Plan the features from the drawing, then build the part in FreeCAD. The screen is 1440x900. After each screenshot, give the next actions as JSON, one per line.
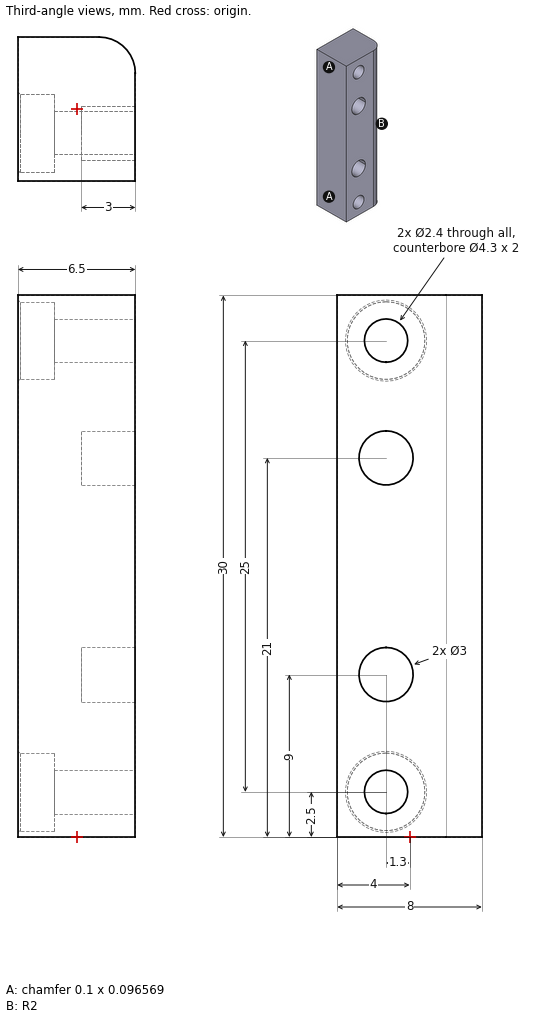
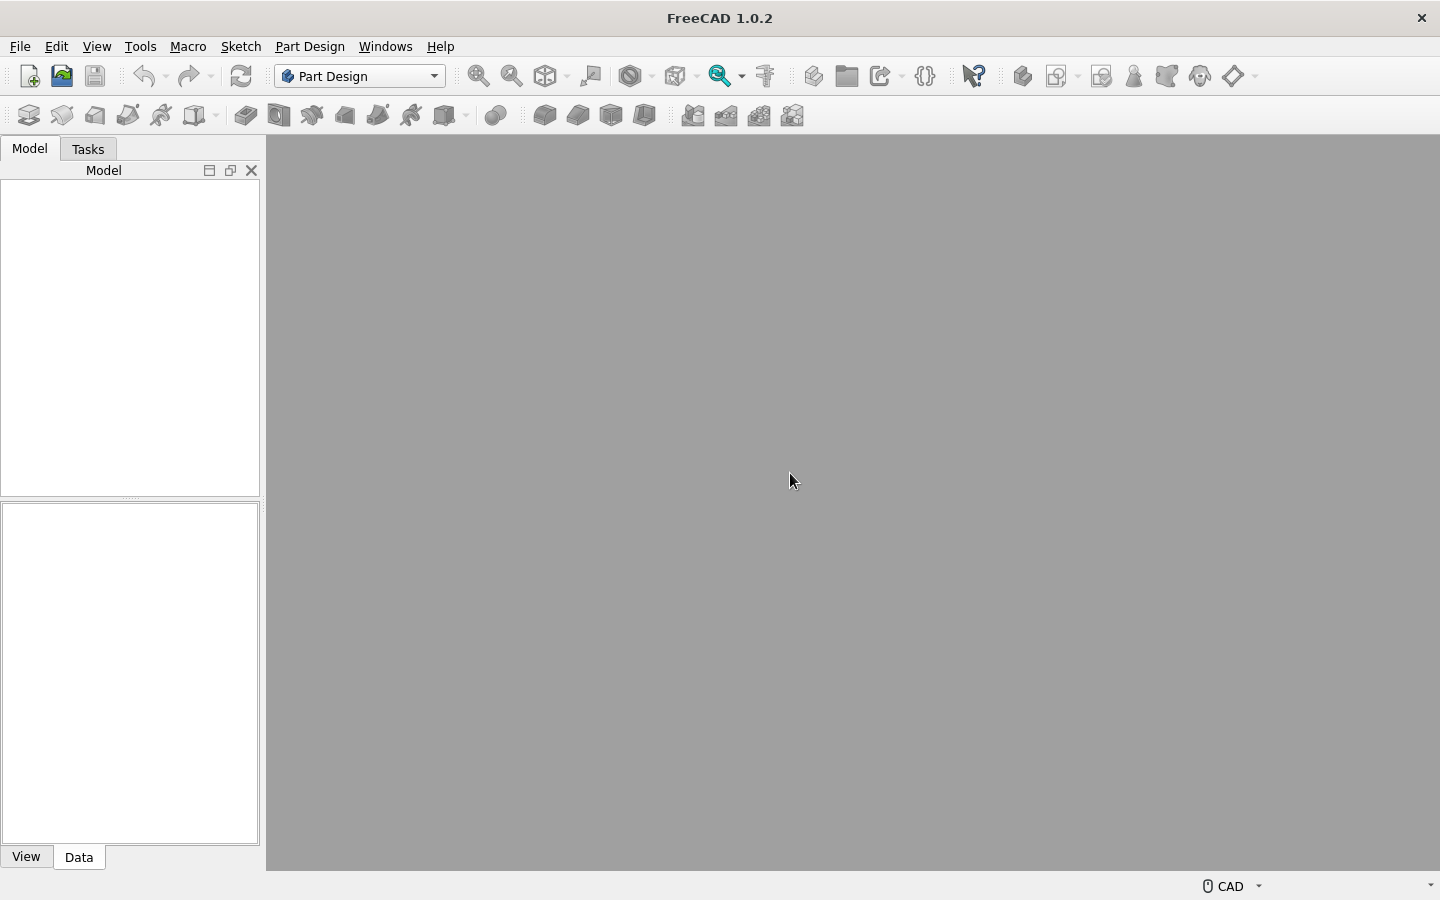
{"action": "left_click", "coordinate": [29, 76]}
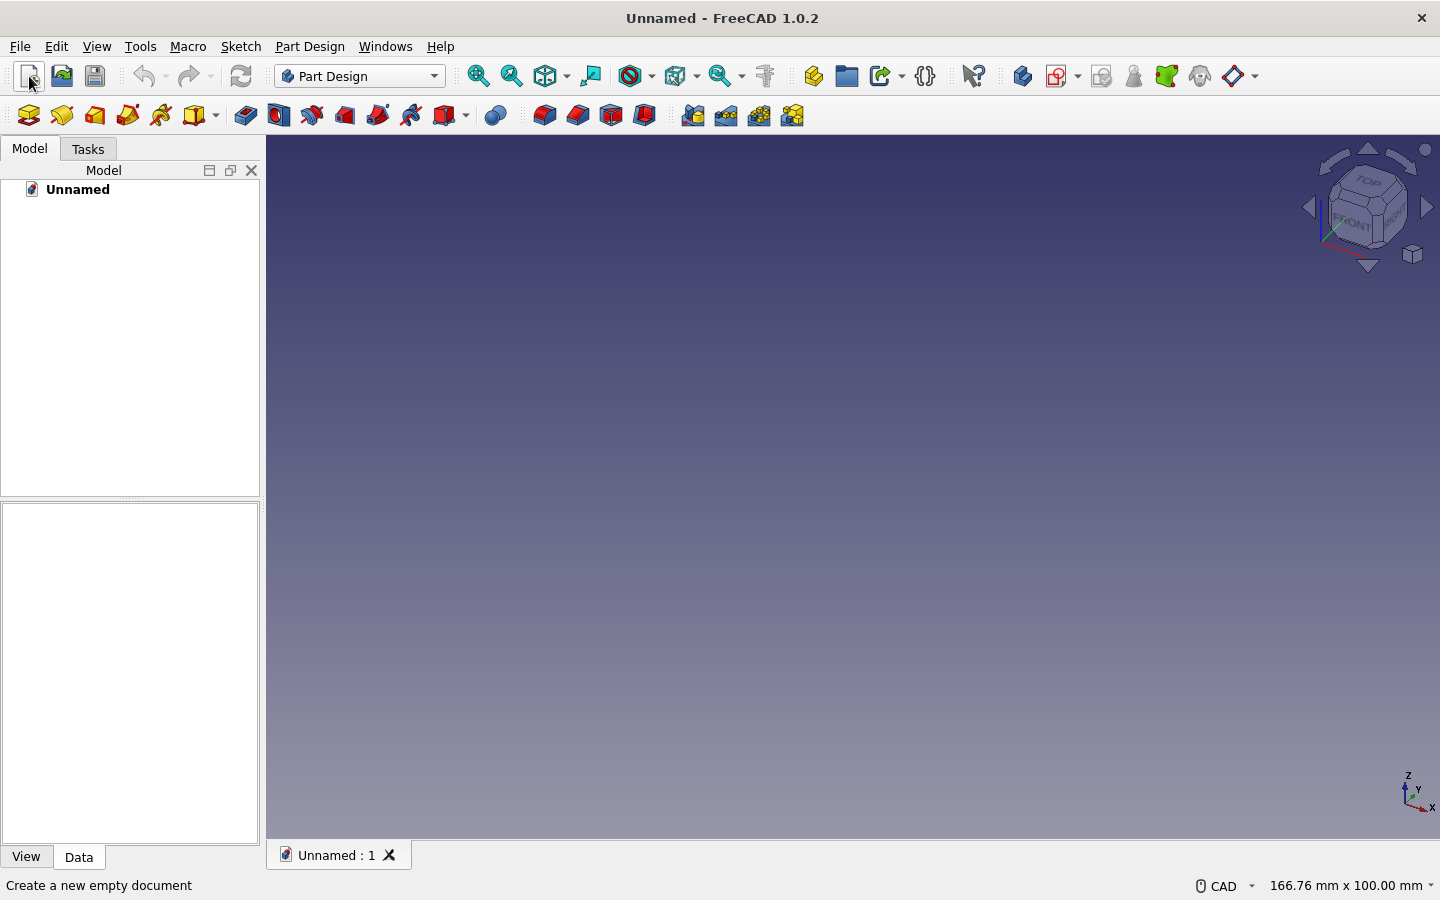
{"action": "left_click", "coordinate": [1023, 76]}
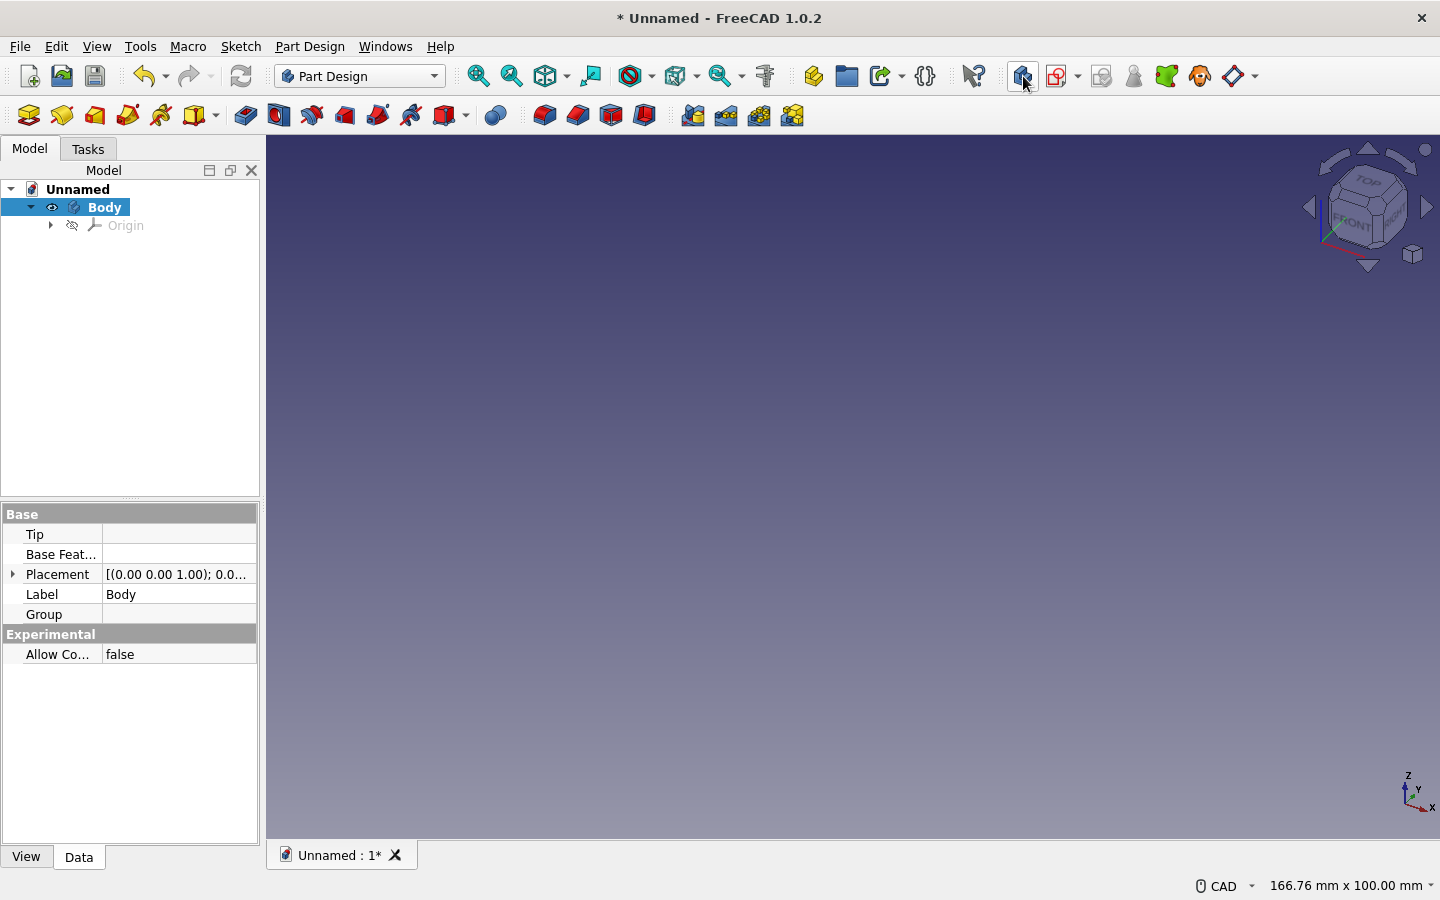
{"action": "left_click", "coordinate": [51, 225]}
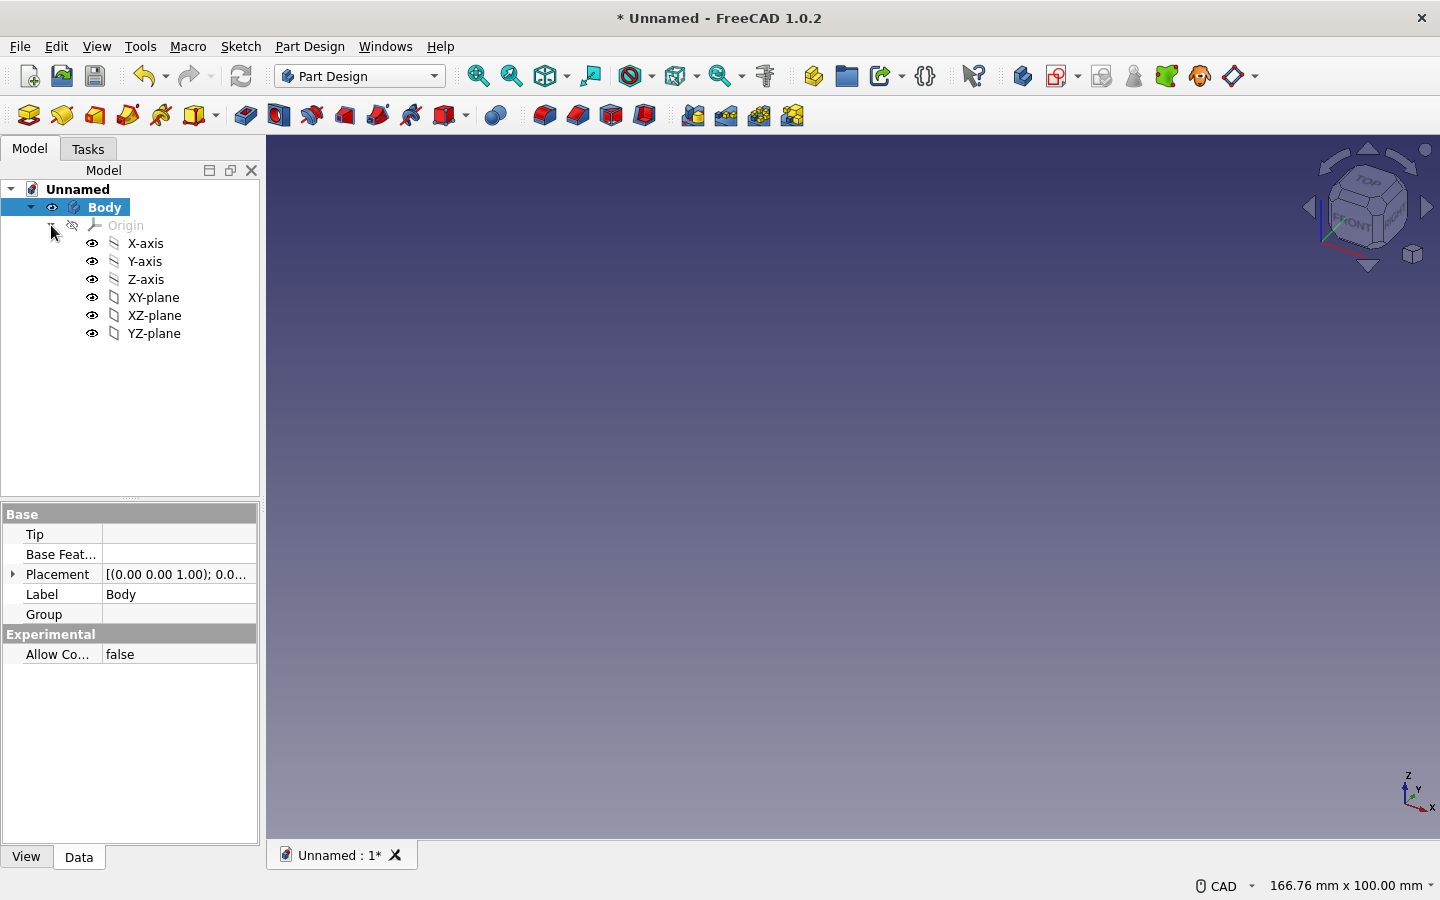
{"action": "left_click", "coordinate": [137, 333]}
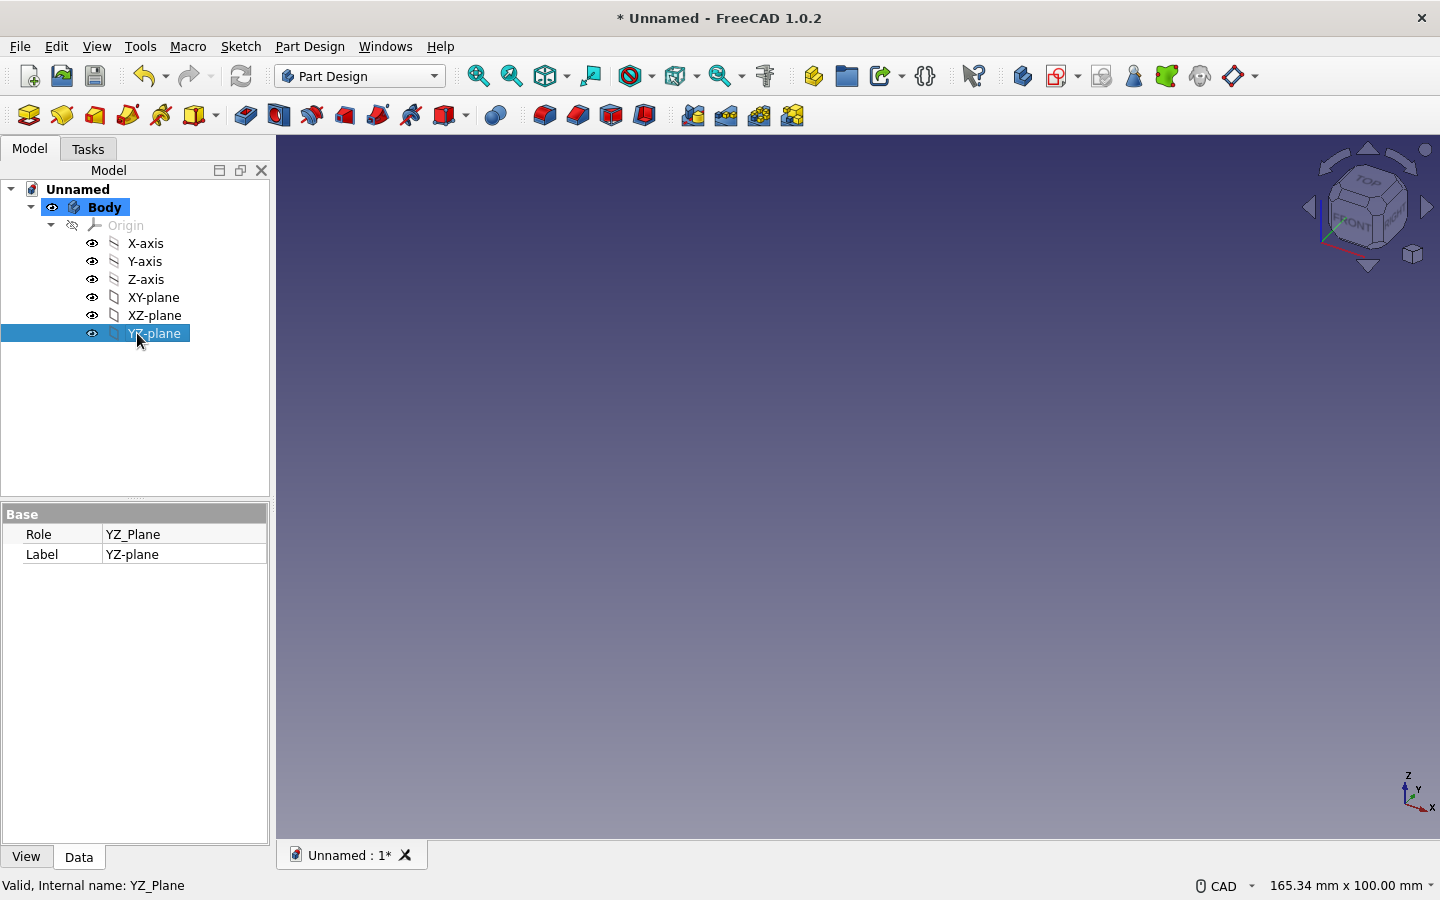
{"action": "left_click", "coordinate": [1232, 76]}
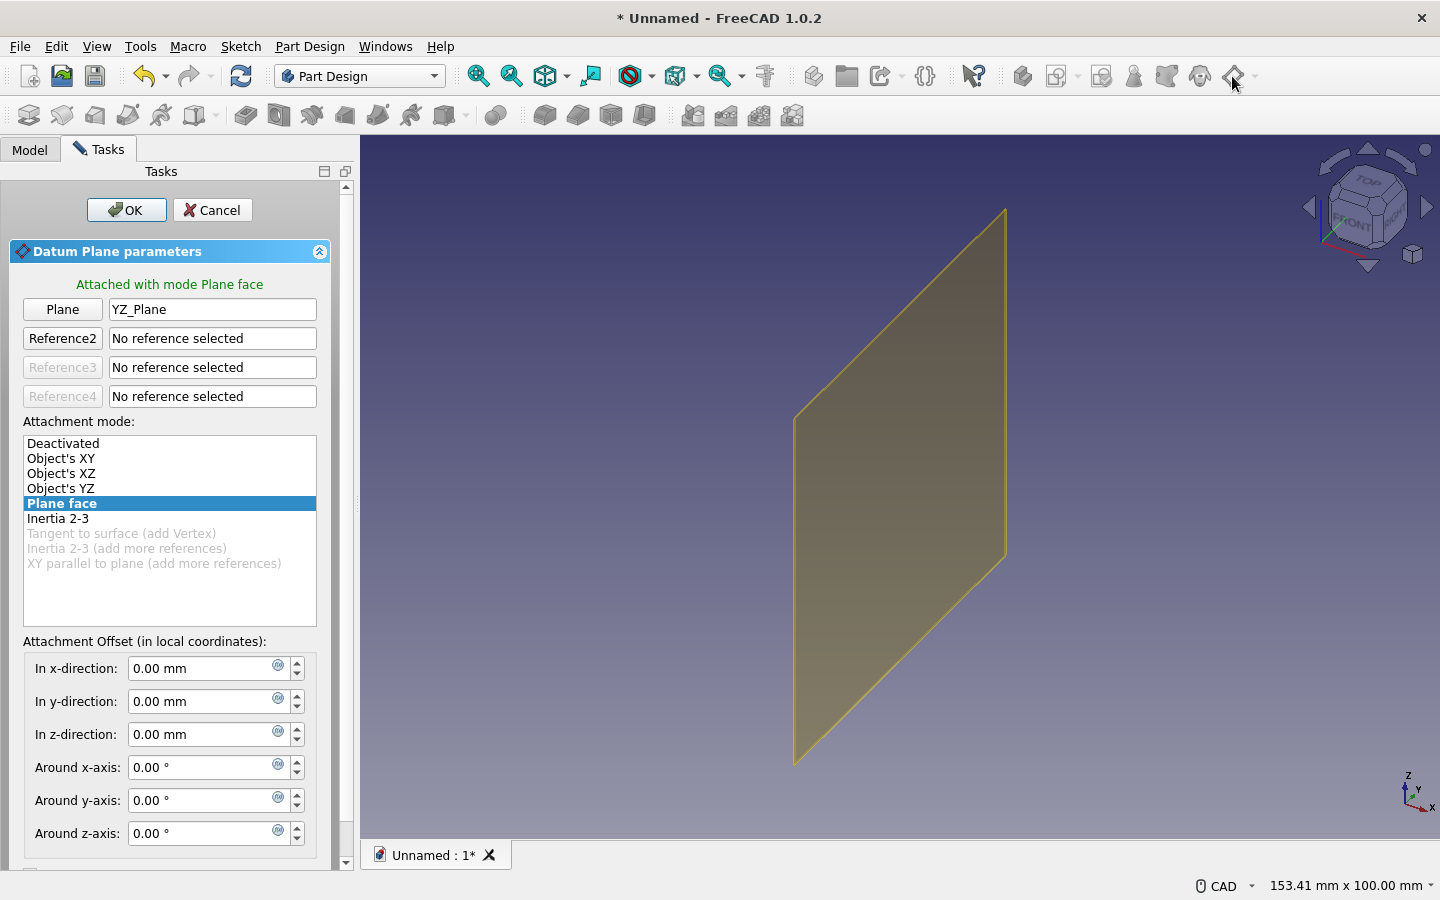
{"action": "triple_click", "coordinate": [210, 734]}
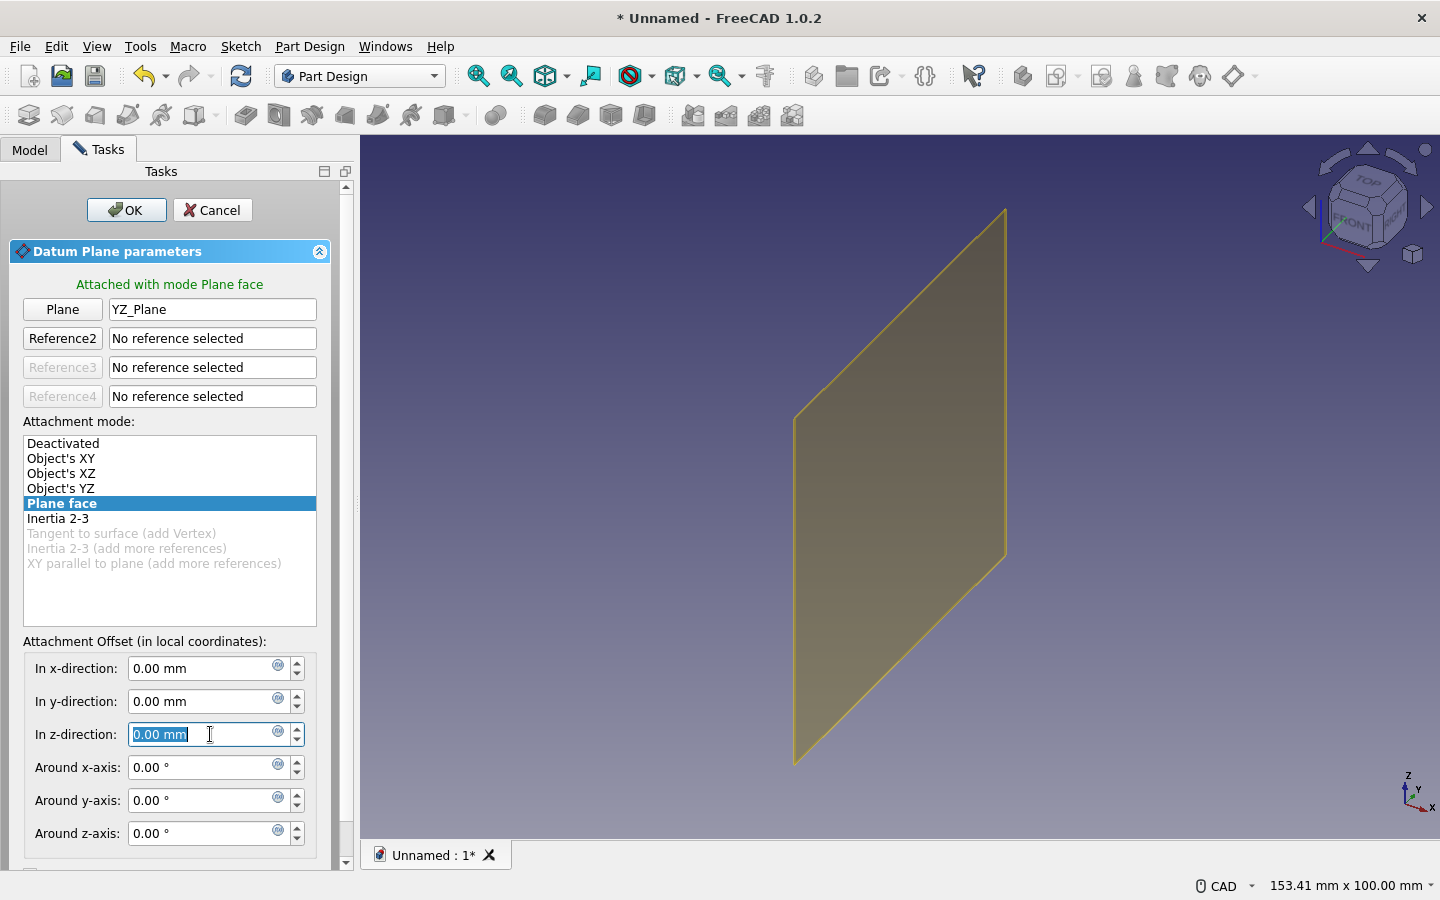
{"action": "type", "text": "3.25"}
{"action": "key", "text": "Tab"}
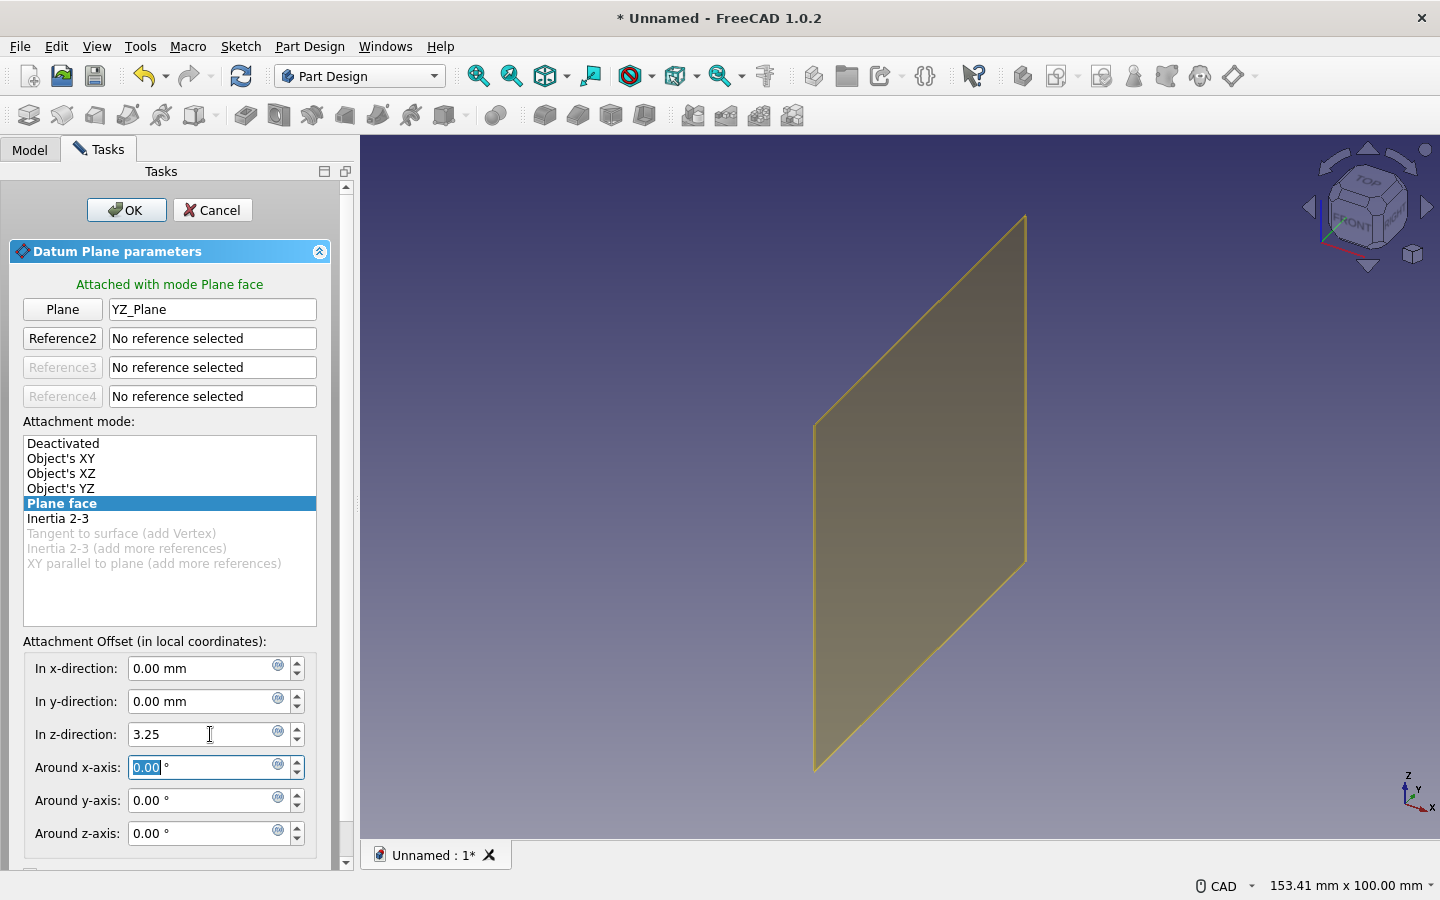
{"action": "left_click", "coordinate": [127, 210]}